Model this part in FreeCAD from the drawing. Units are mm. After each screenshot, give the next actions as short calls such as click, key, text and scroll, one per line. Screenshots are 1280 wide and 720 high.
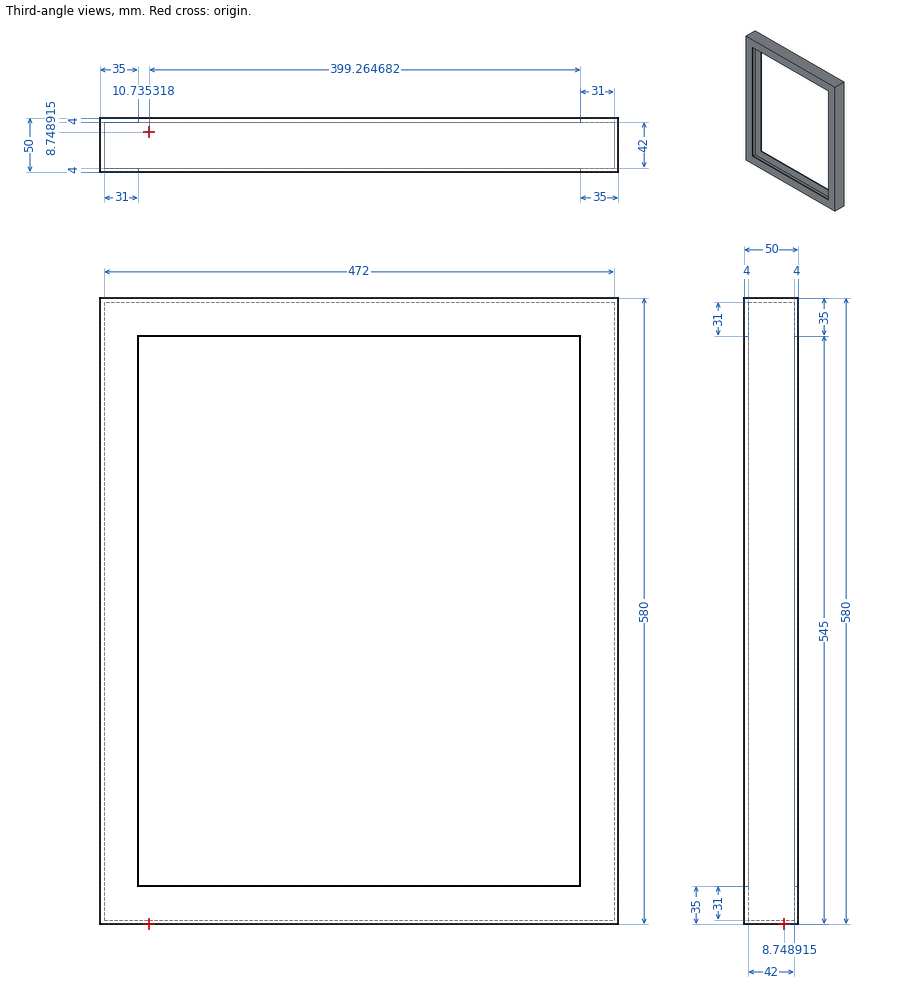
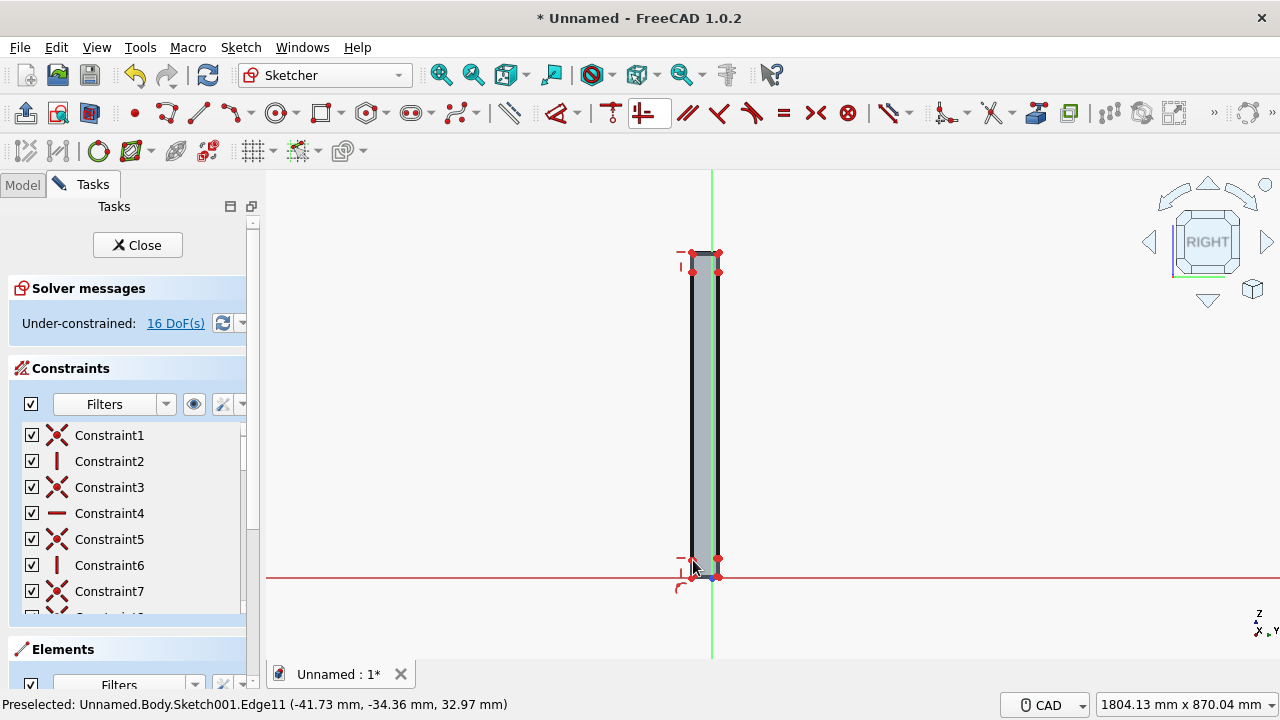
scroll(711, 577, up, 14)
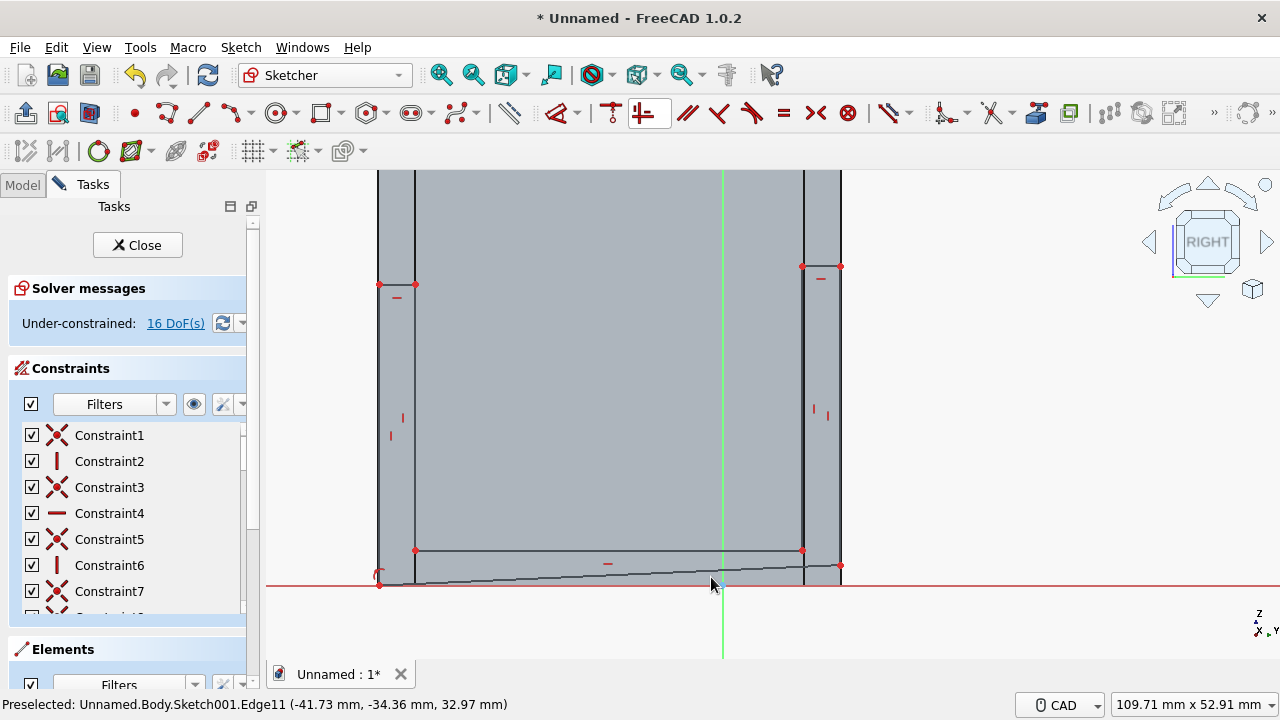
click(702, 571)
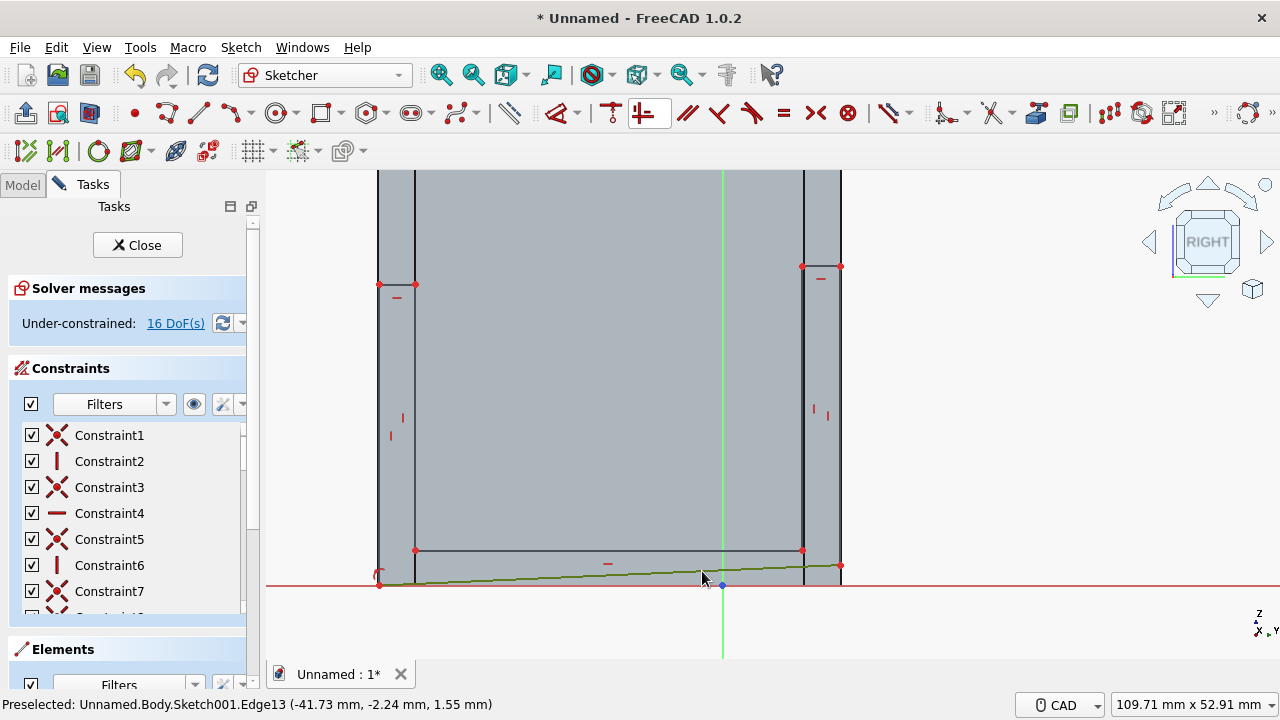
click(666, 114)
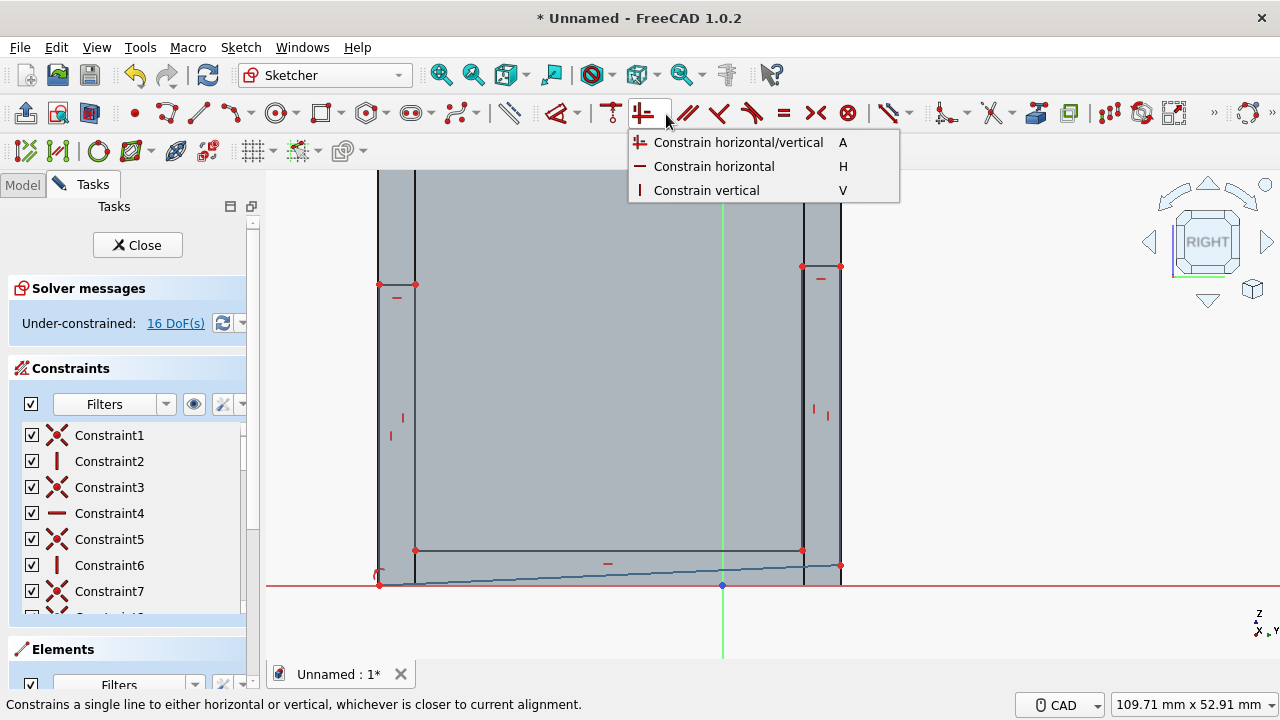
click(764, 166)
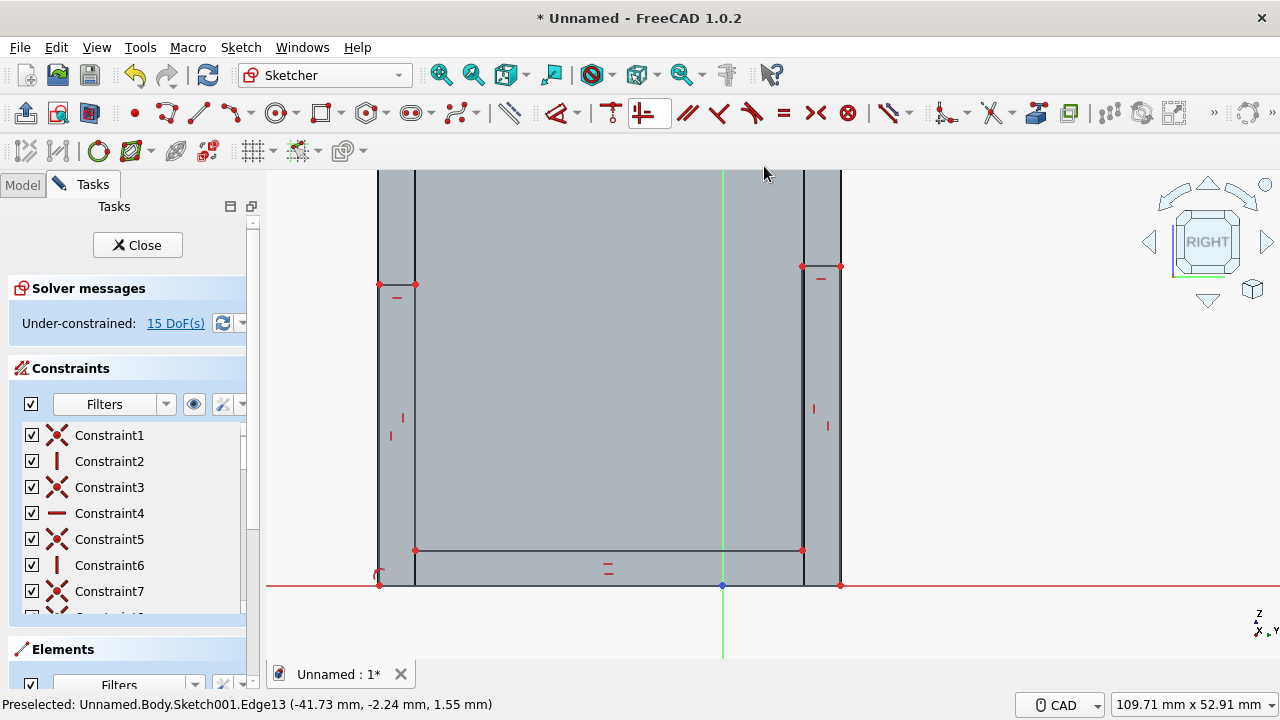
click(556, 114)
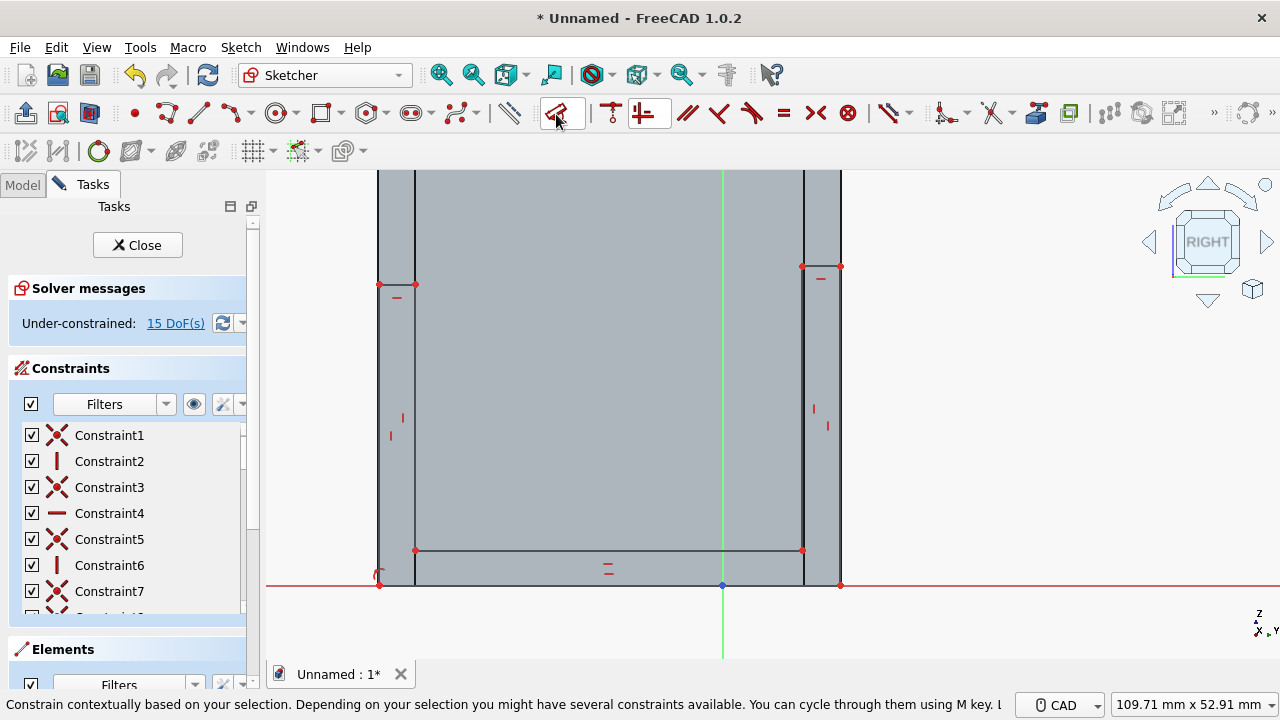
scroll(711, 577, down, 14)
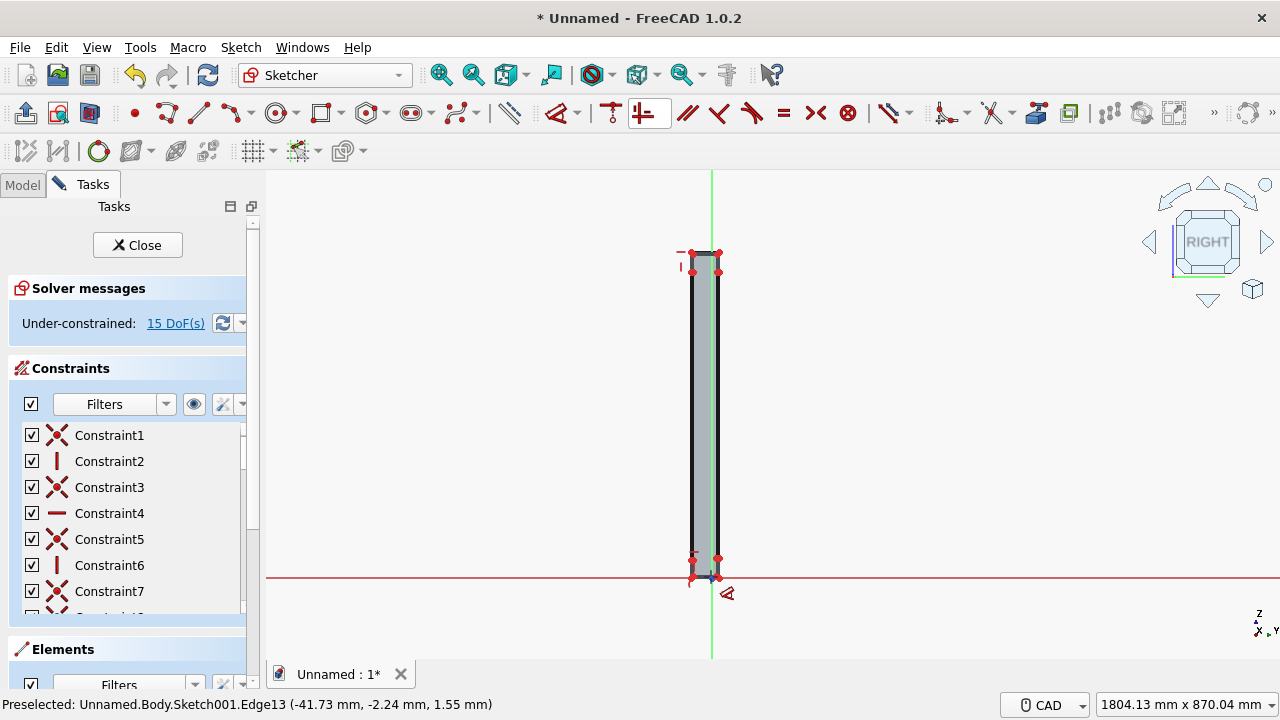
scroll(718, 272, up, 15)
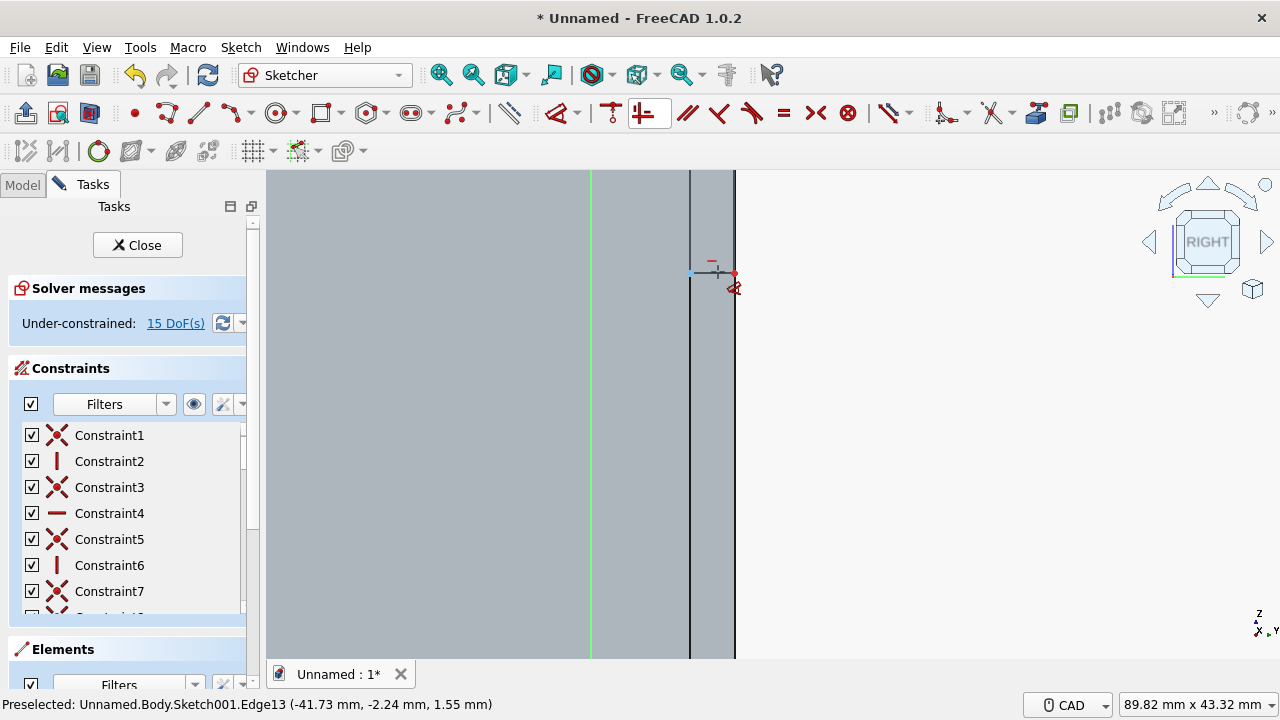
click(703, 273)
click(712, 239)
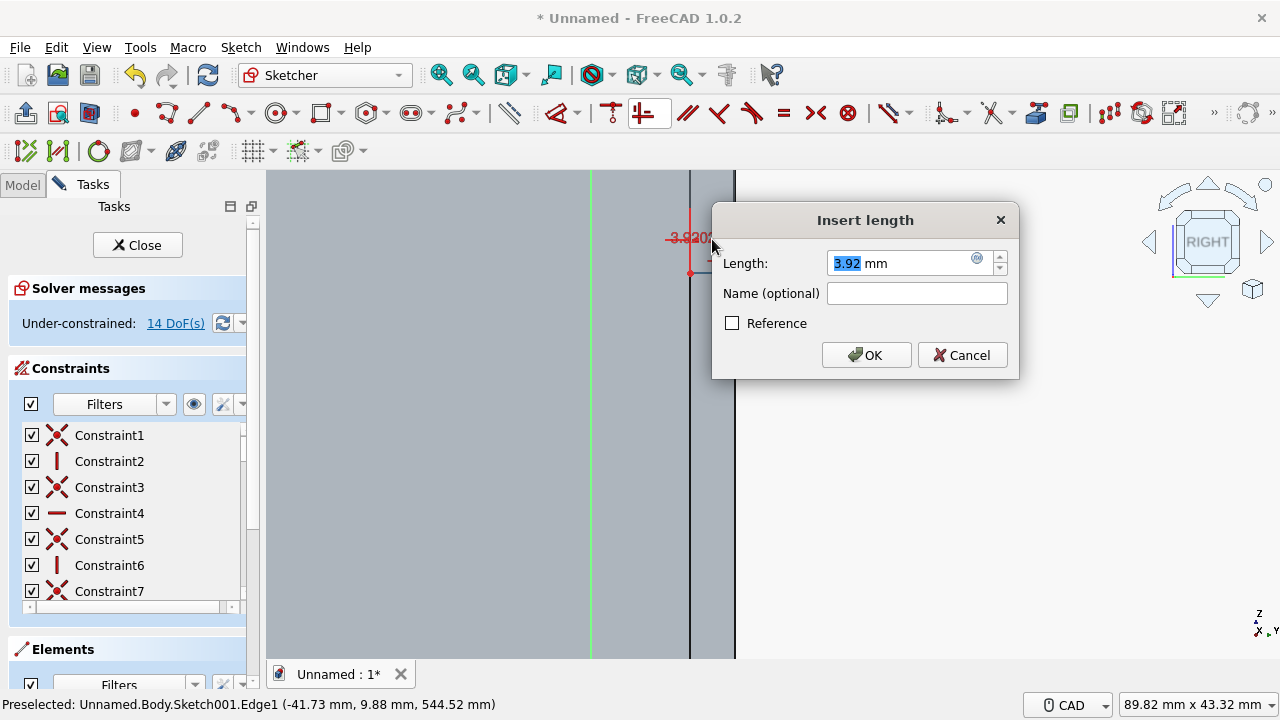
text(4)
key(Return)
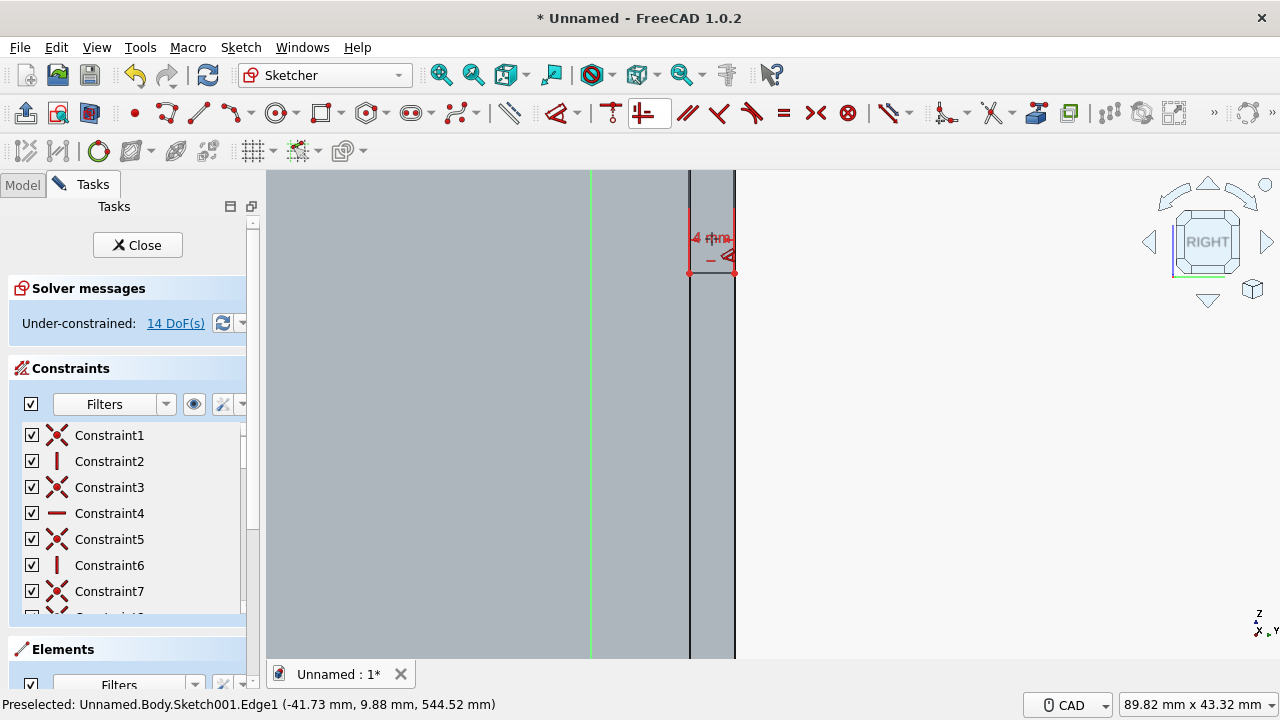
scroll(718, 271, down, 15)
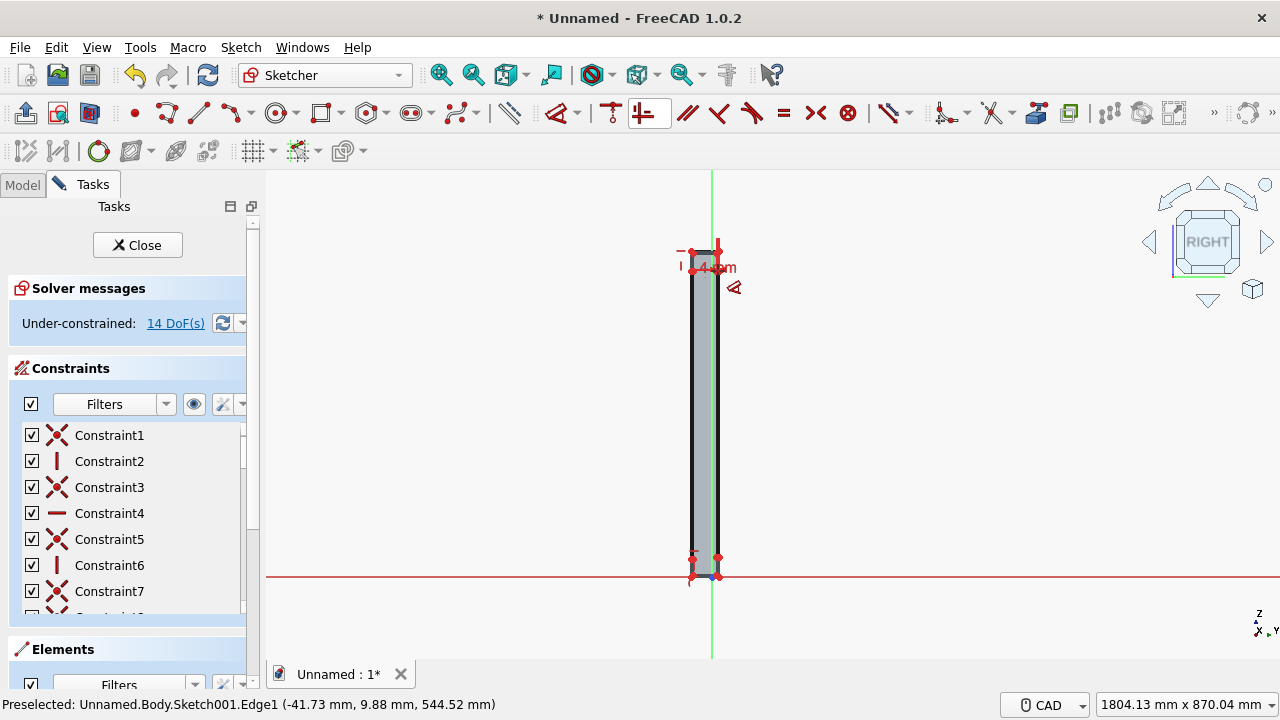
scroll(692, 271, up, 15)